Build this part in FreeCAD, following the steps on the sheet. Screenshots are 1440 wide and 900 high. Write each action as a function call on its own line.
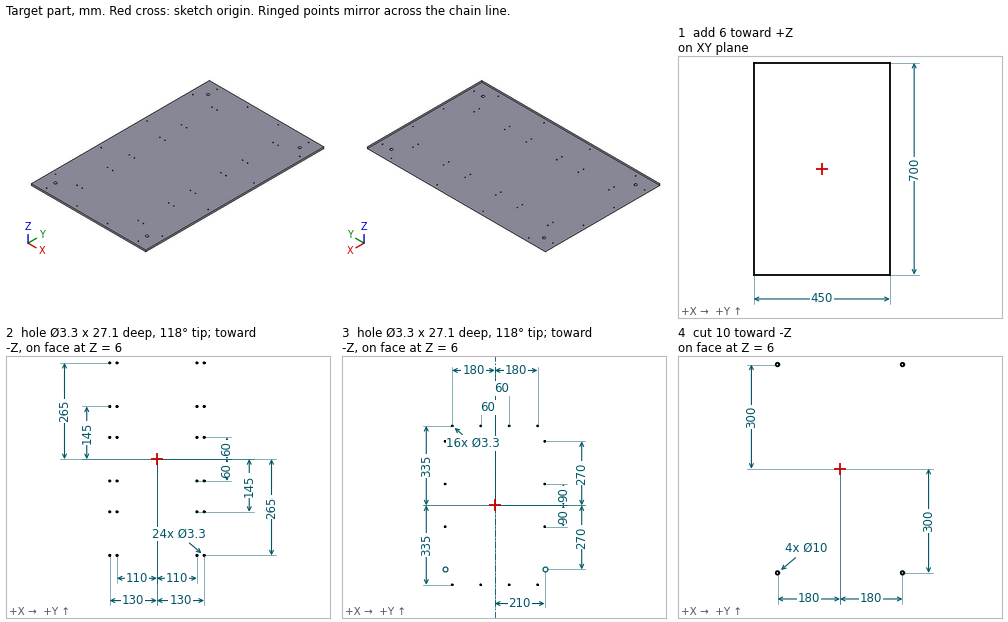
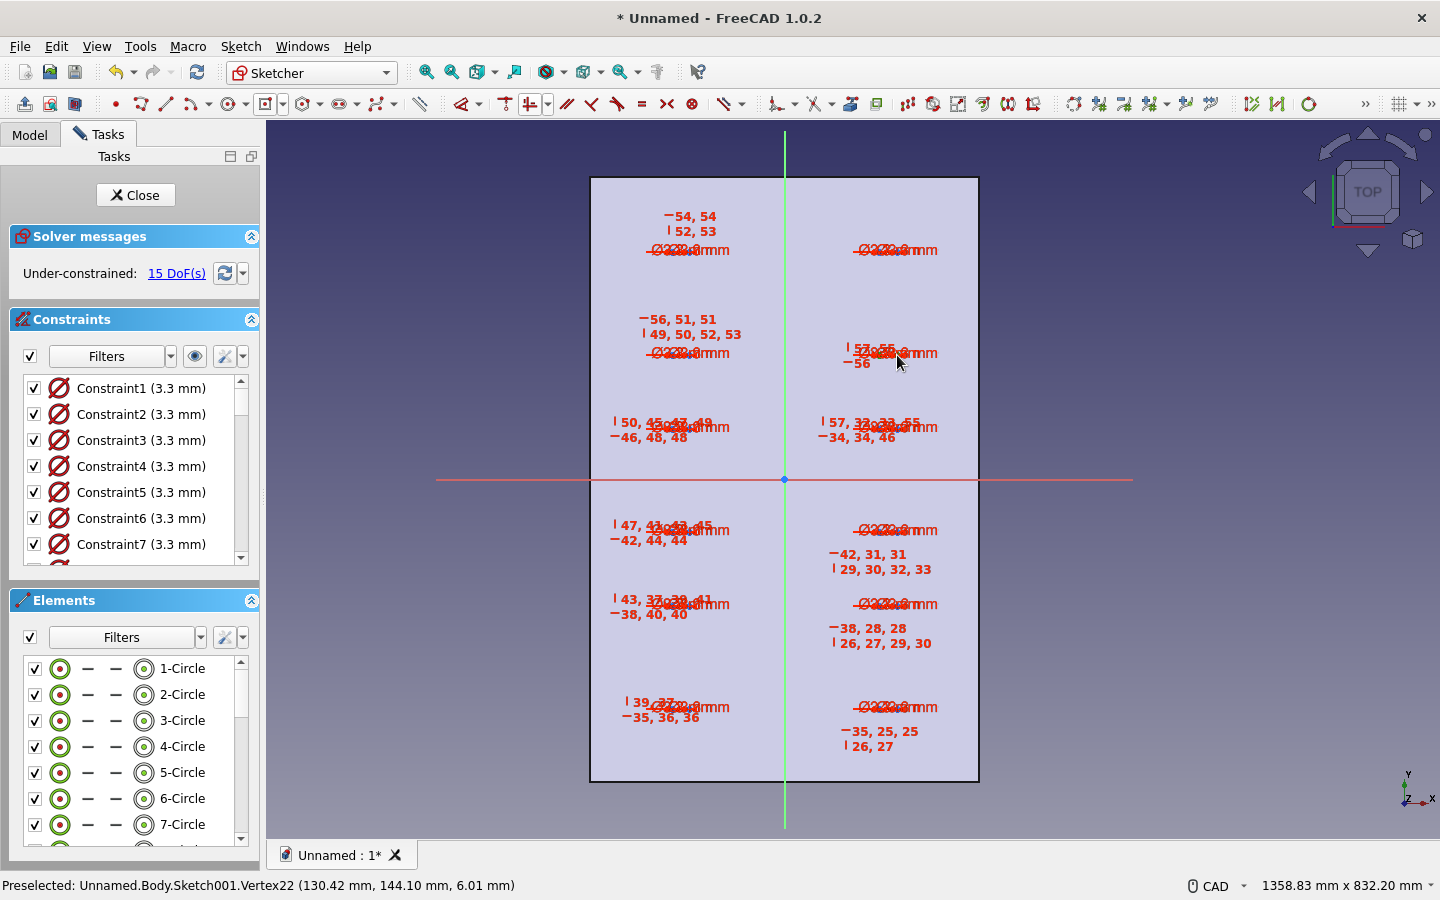
click(548, 104)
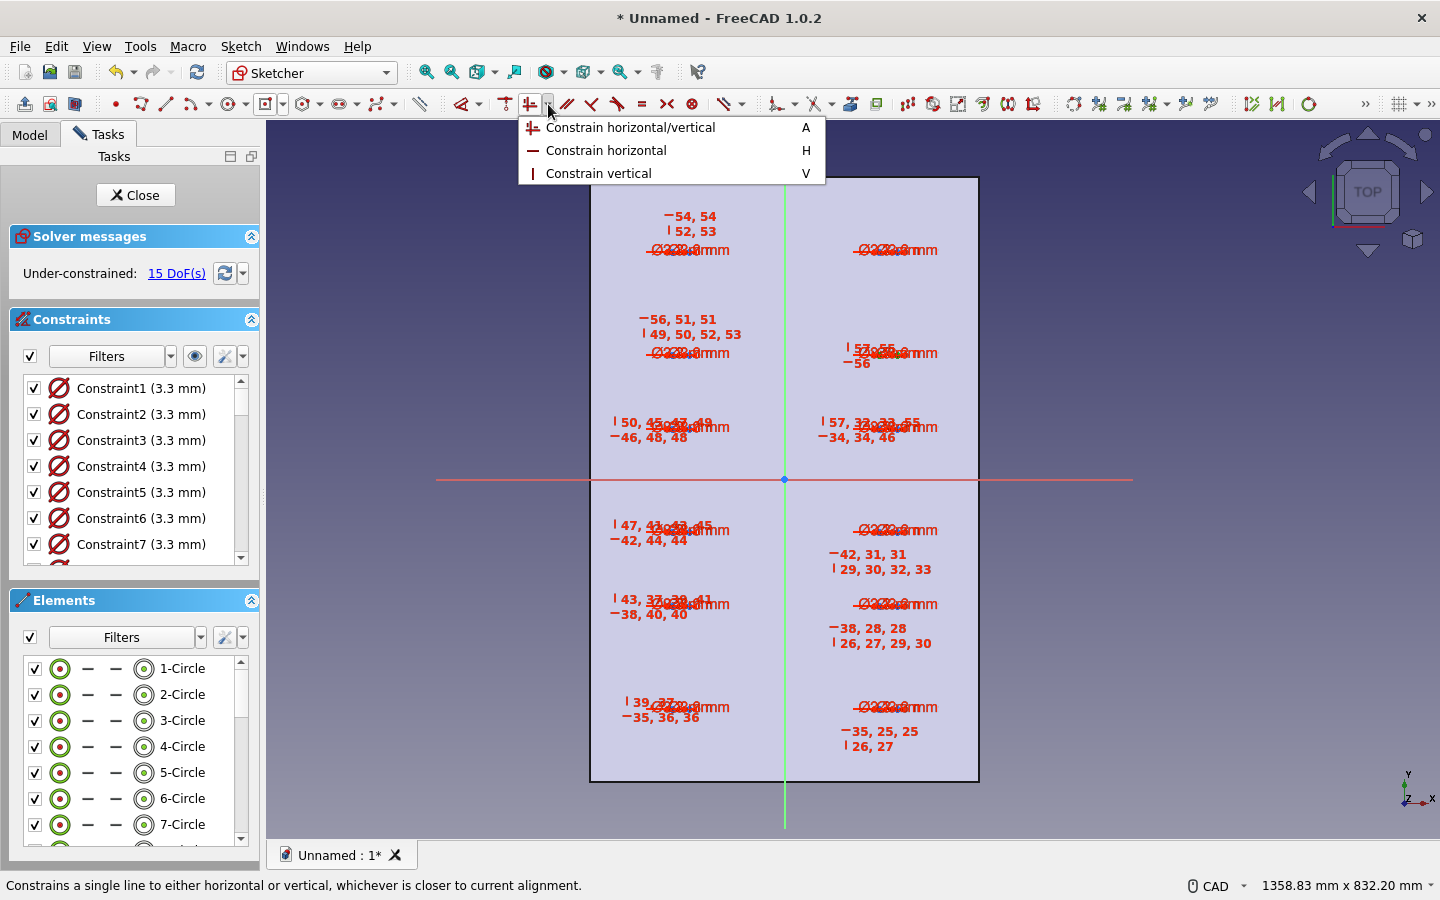
click(672, 150)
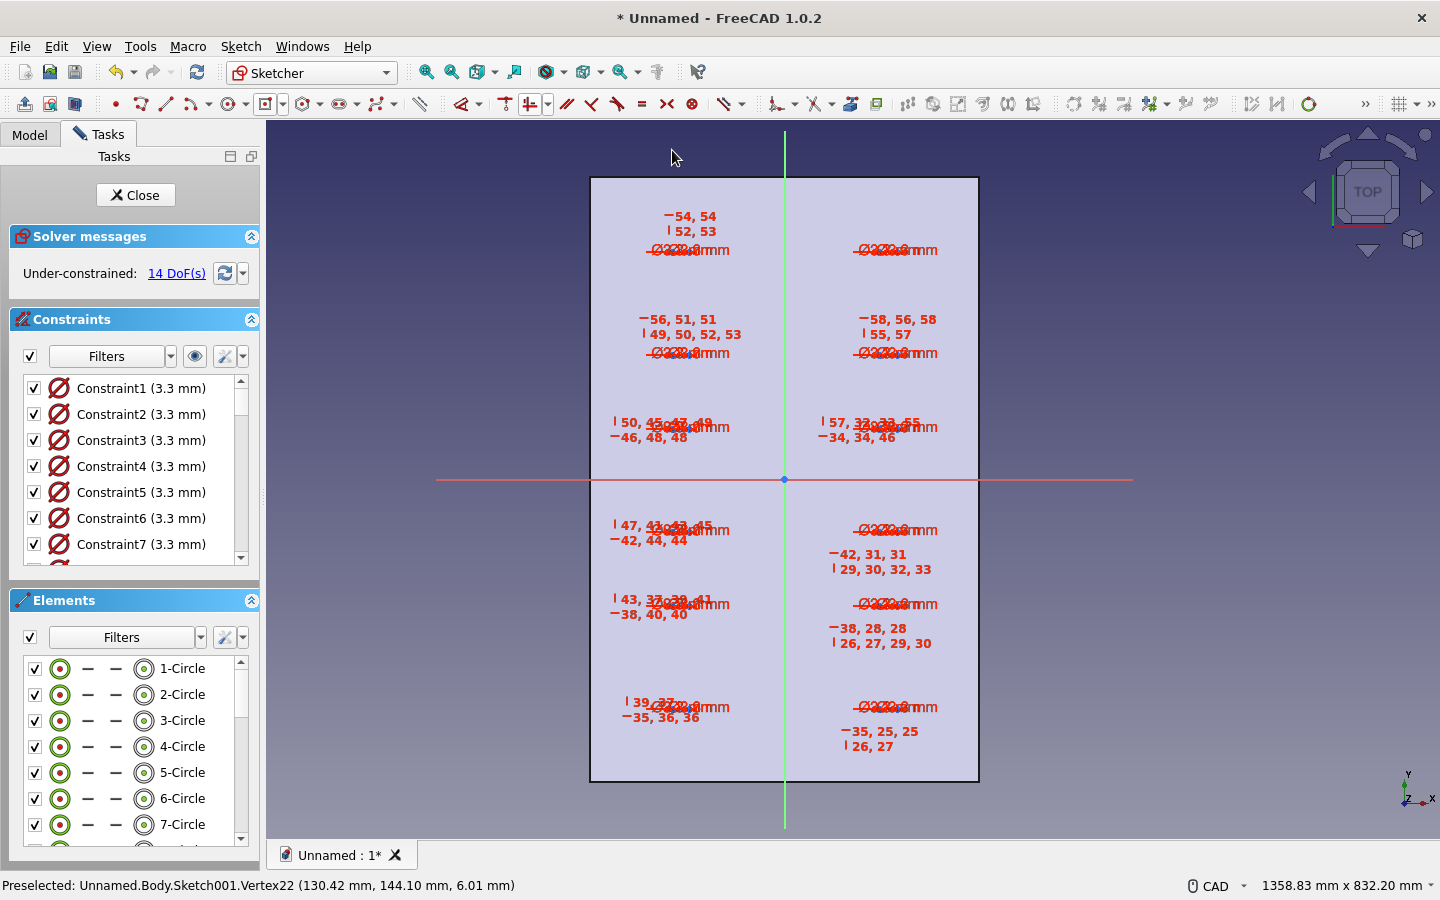
click(879, 355)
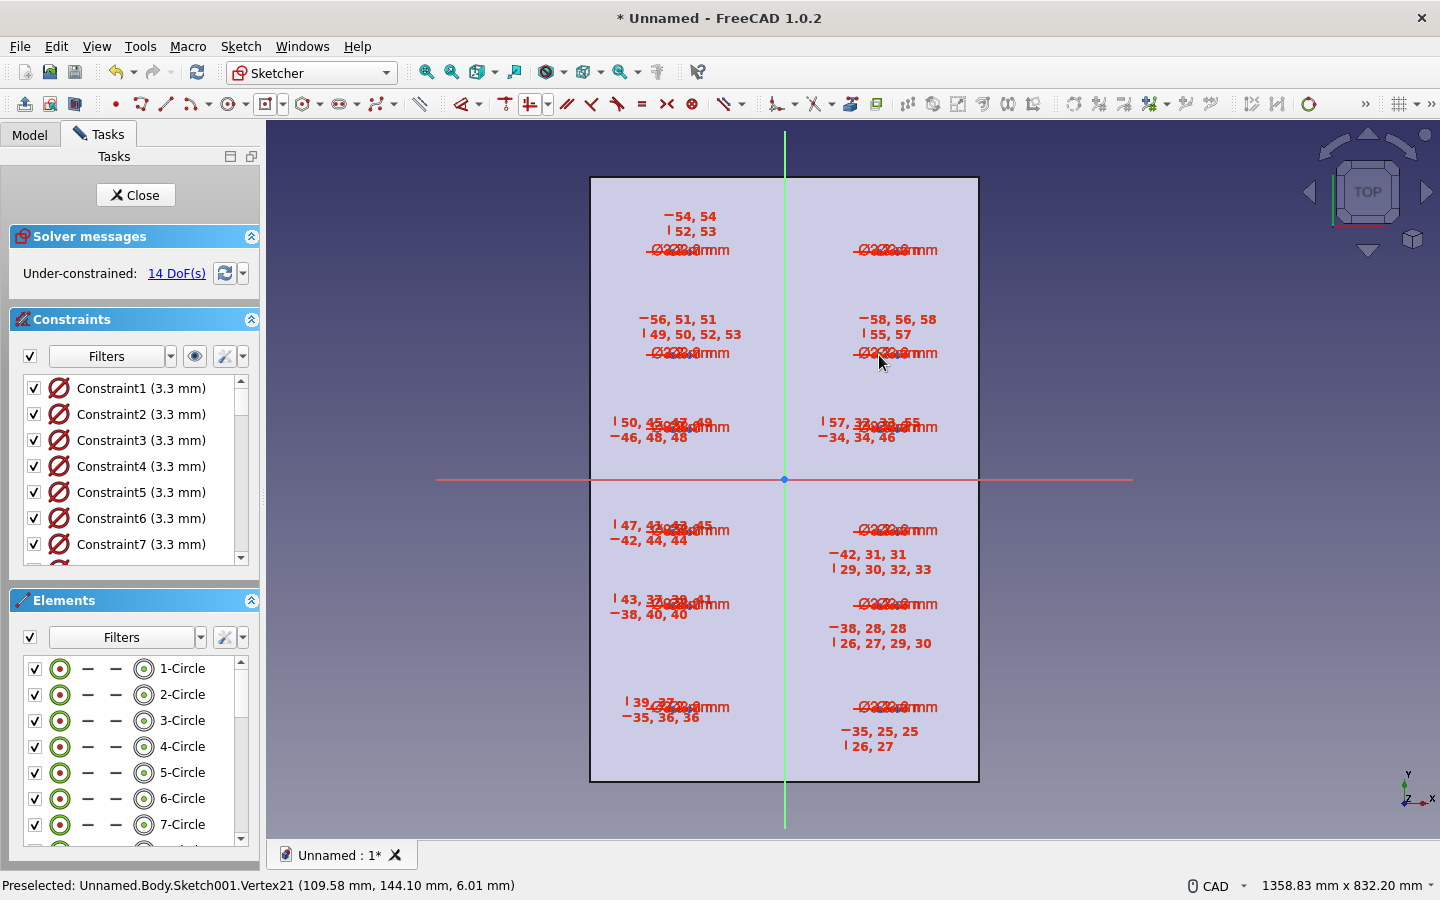
click(879, 252)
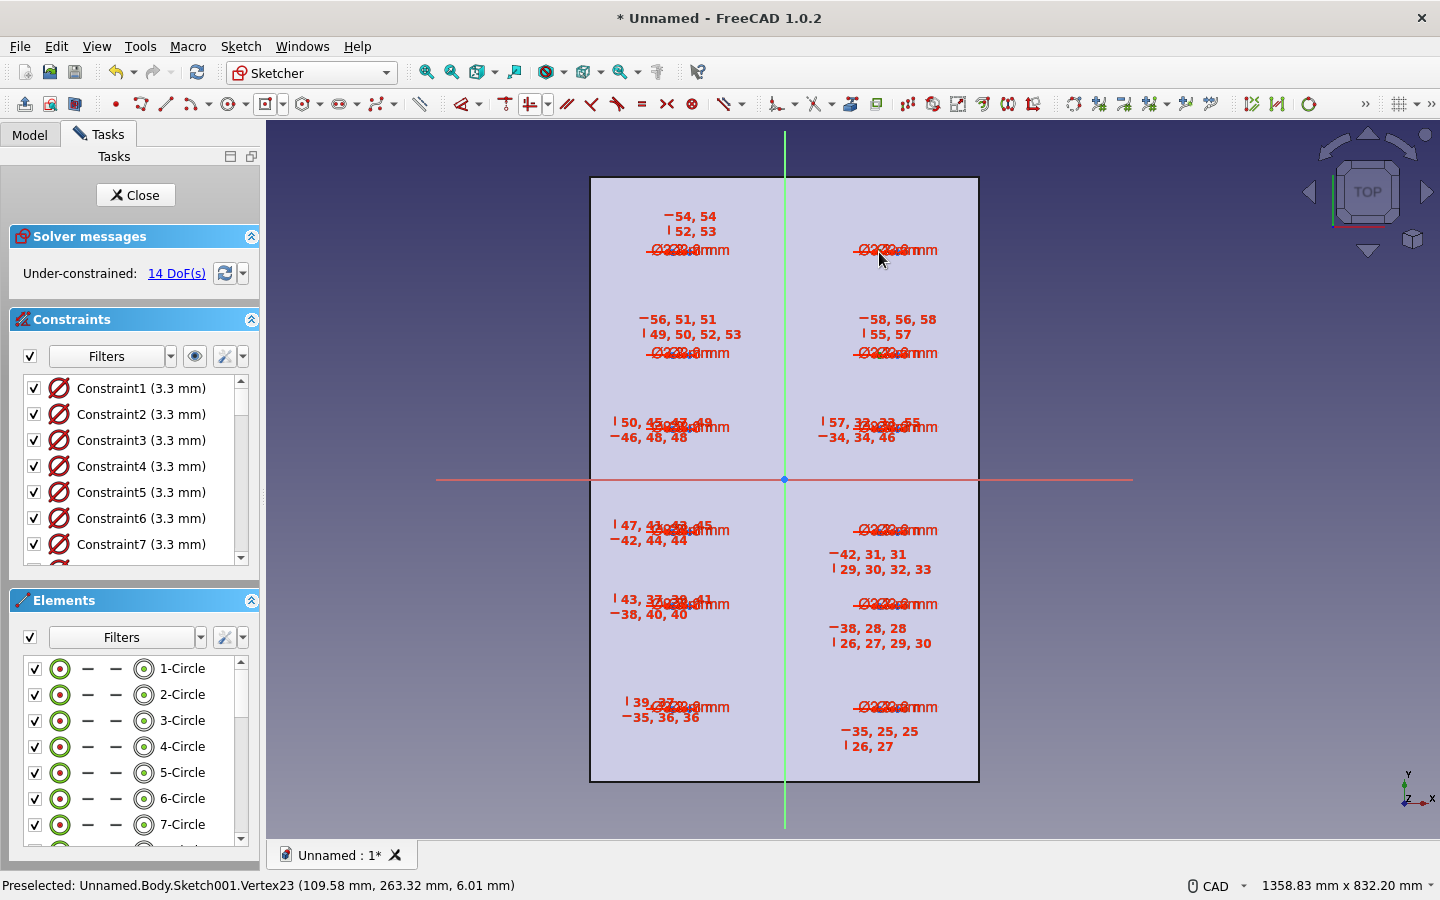
key(v)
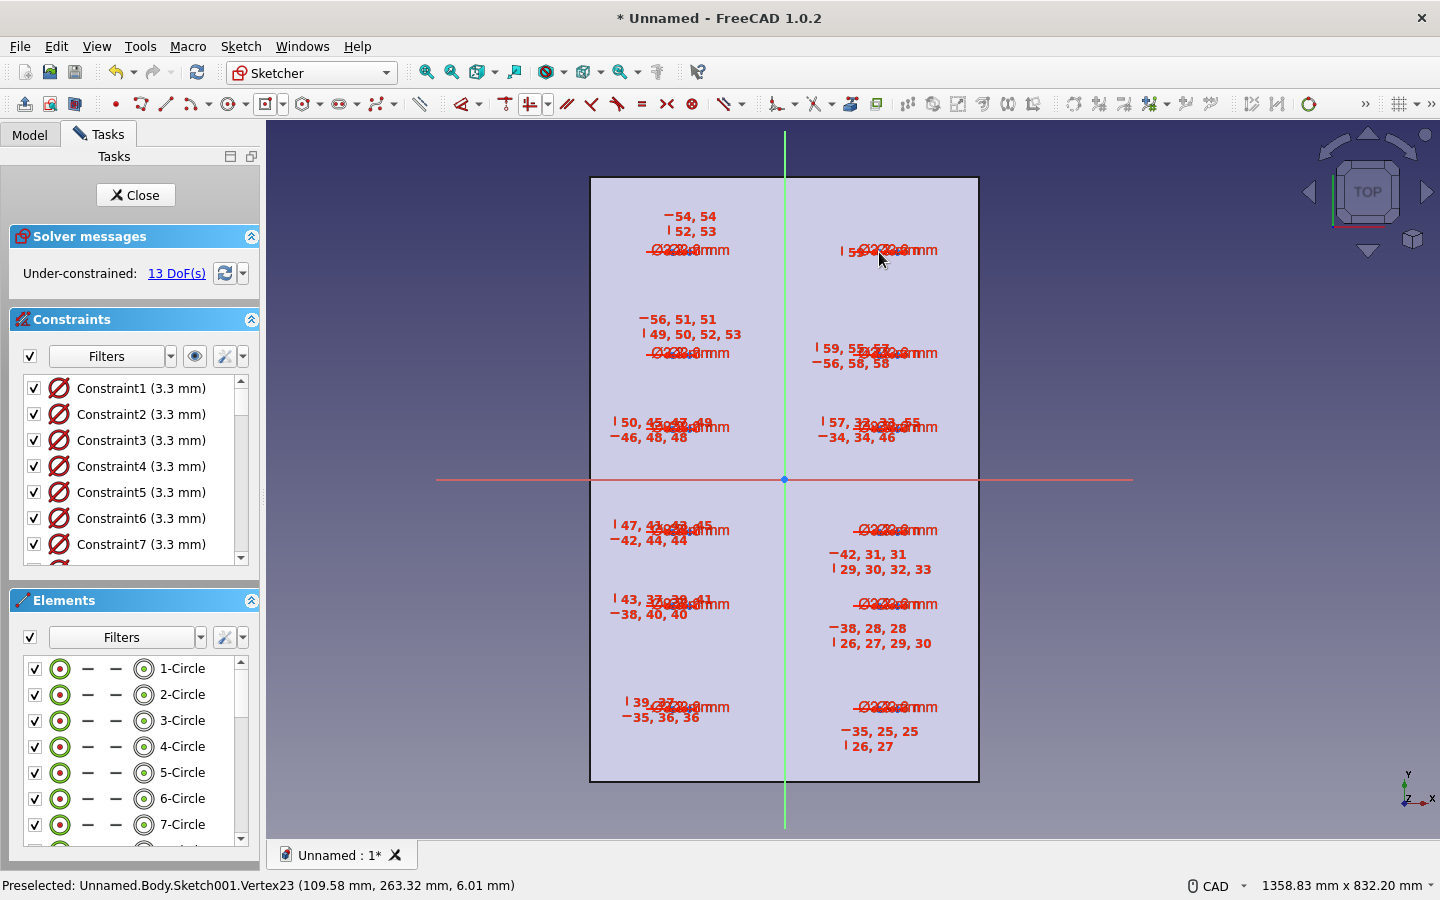
click(689, 252)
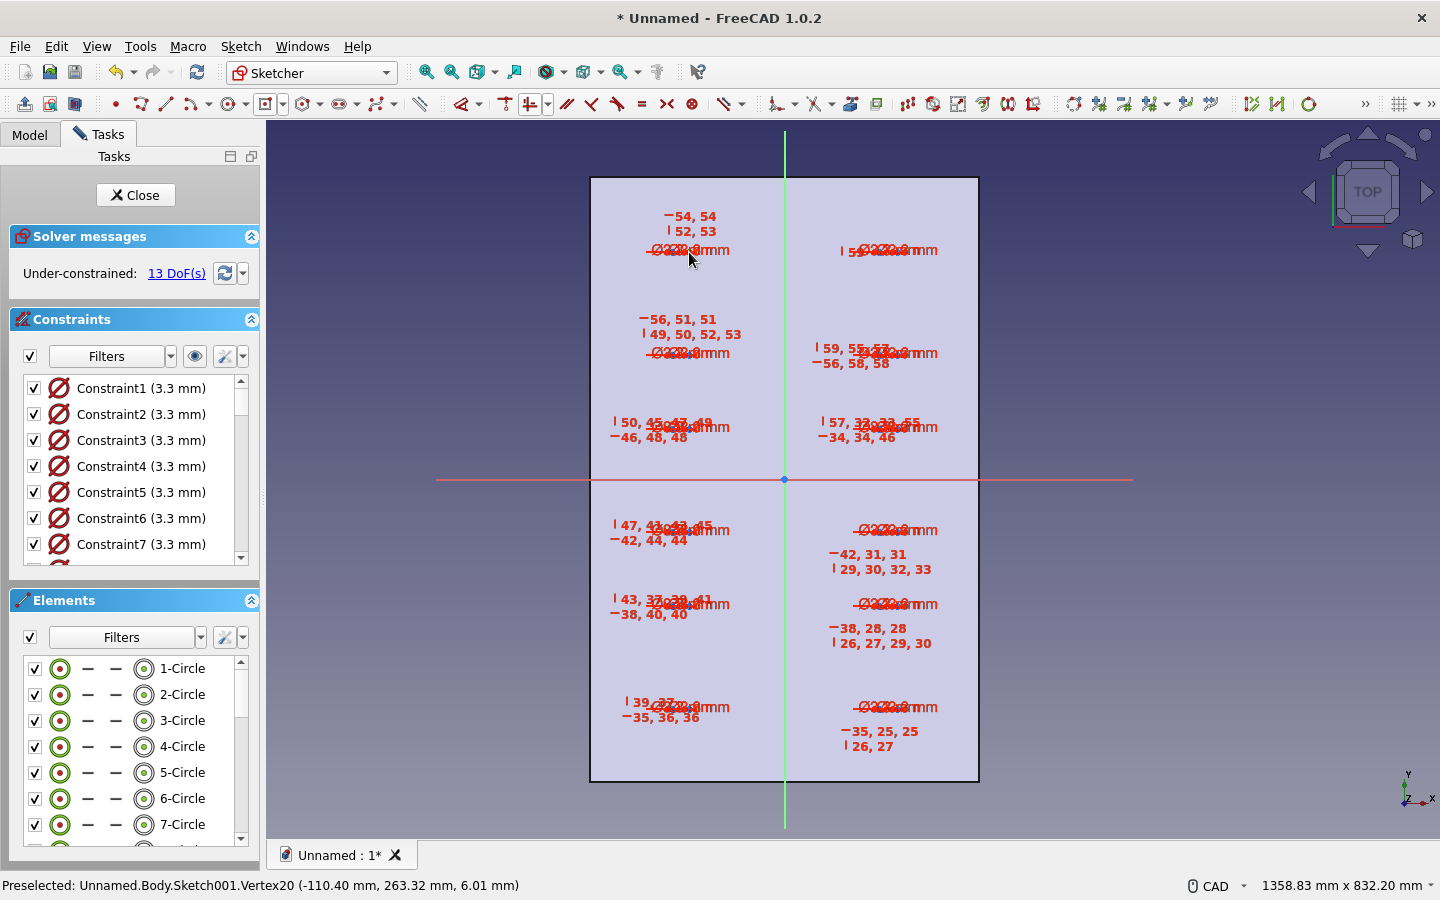
click(879, 252)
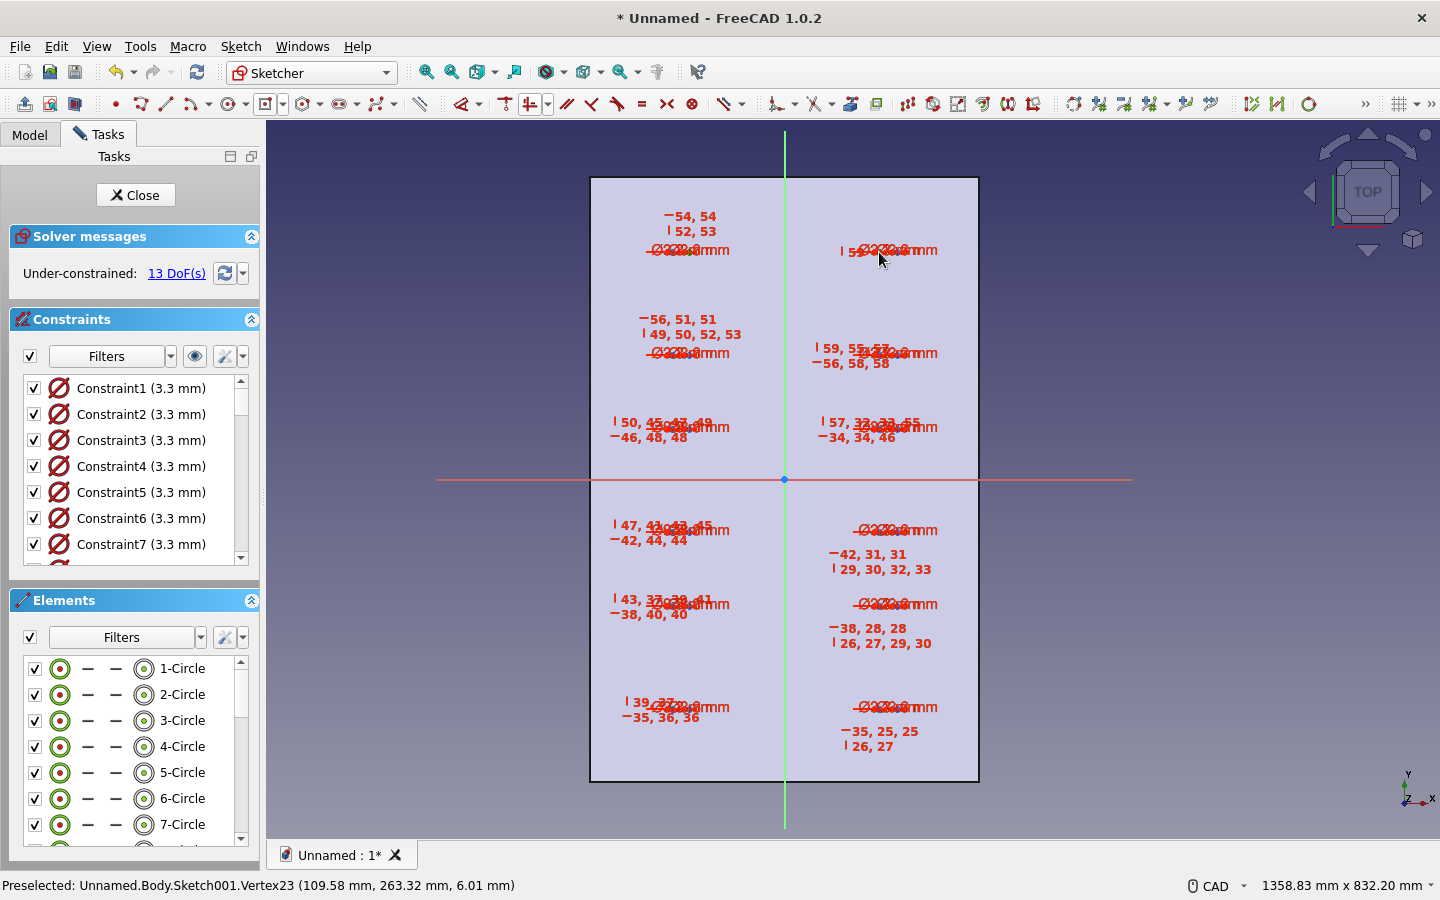
click(548, 104)